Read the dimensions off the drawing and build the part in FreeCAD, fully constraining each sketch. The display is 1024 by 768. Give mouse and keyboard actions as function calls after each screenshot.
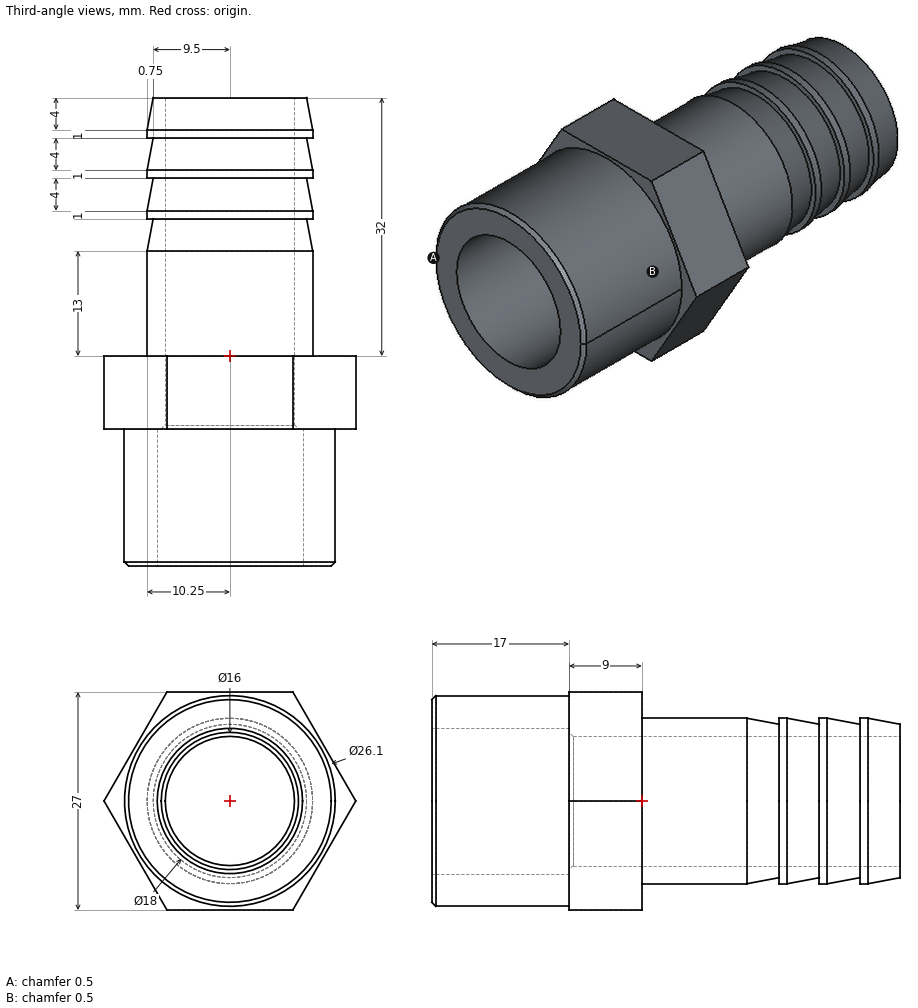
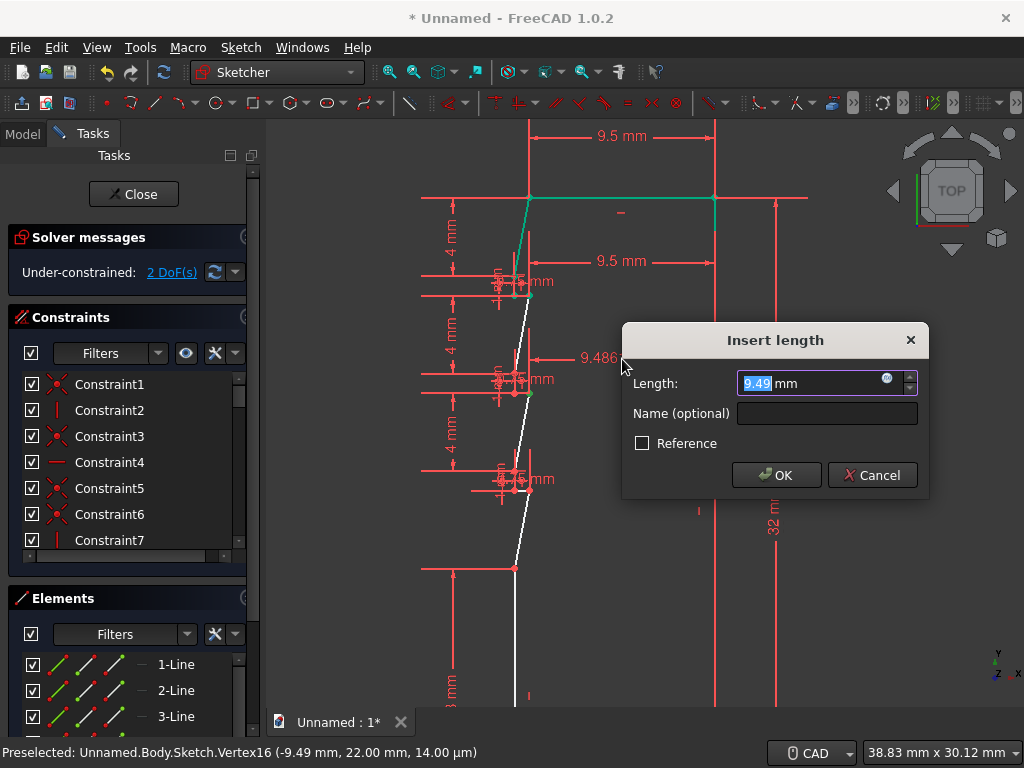
text(9.5)
key(Return)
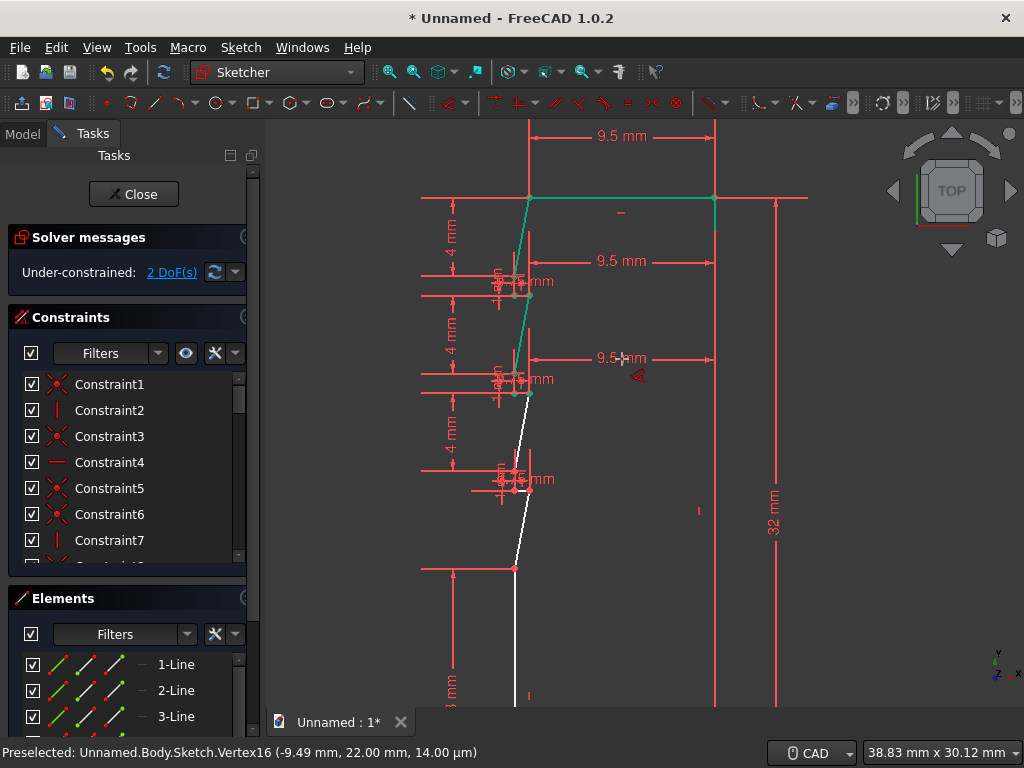
click(530, 491)
click(622, 457)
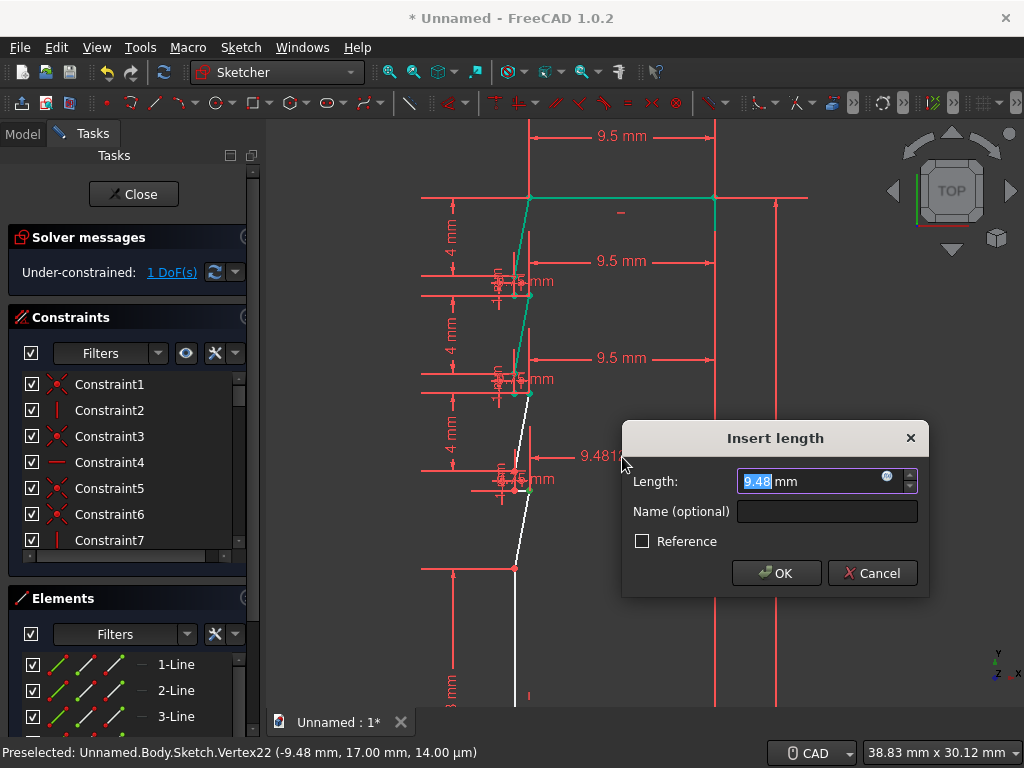
text(9.5)
key(Return)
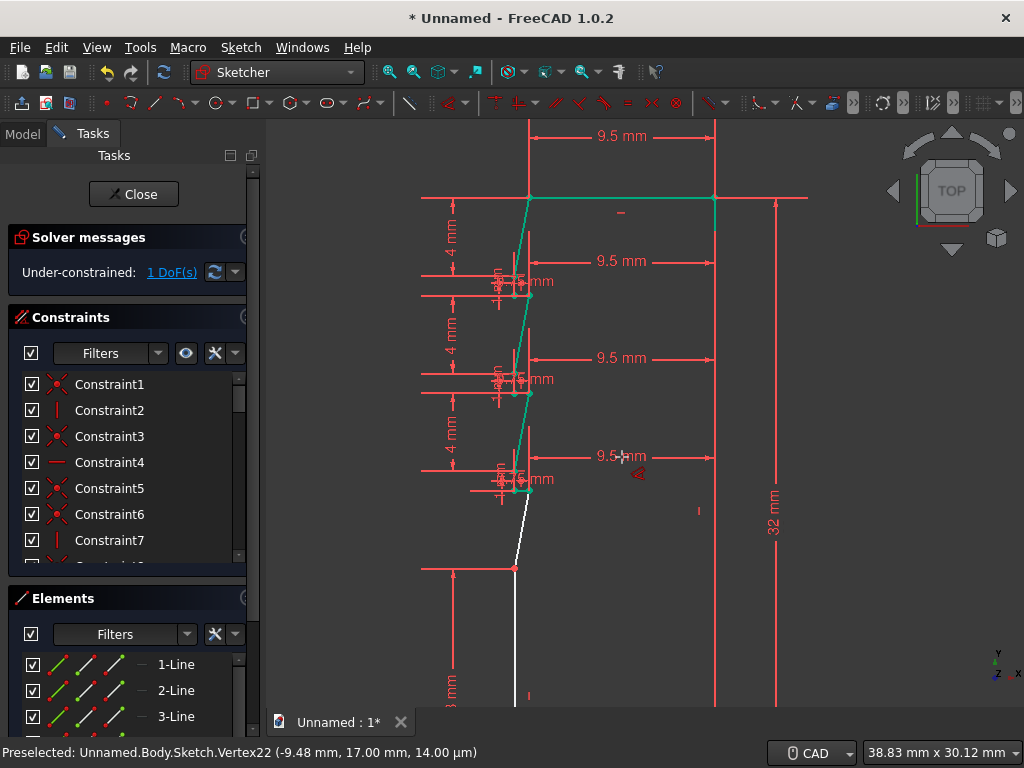
scroll(530, 295, down, 3)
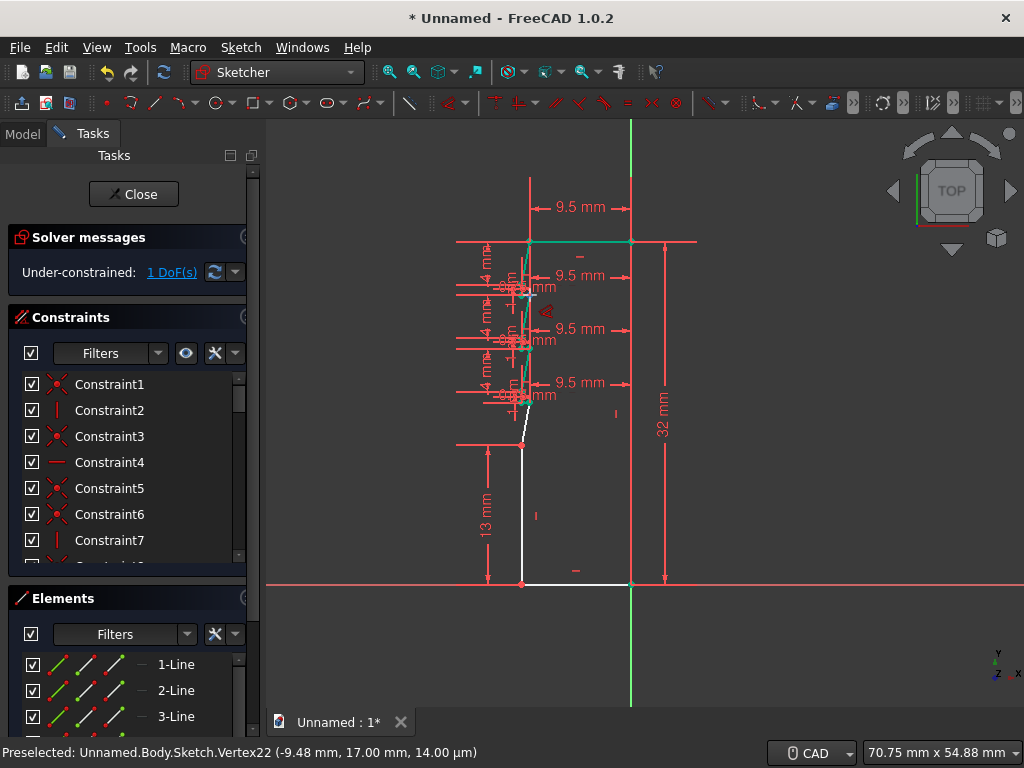
click(555, 585)
click(577, 619)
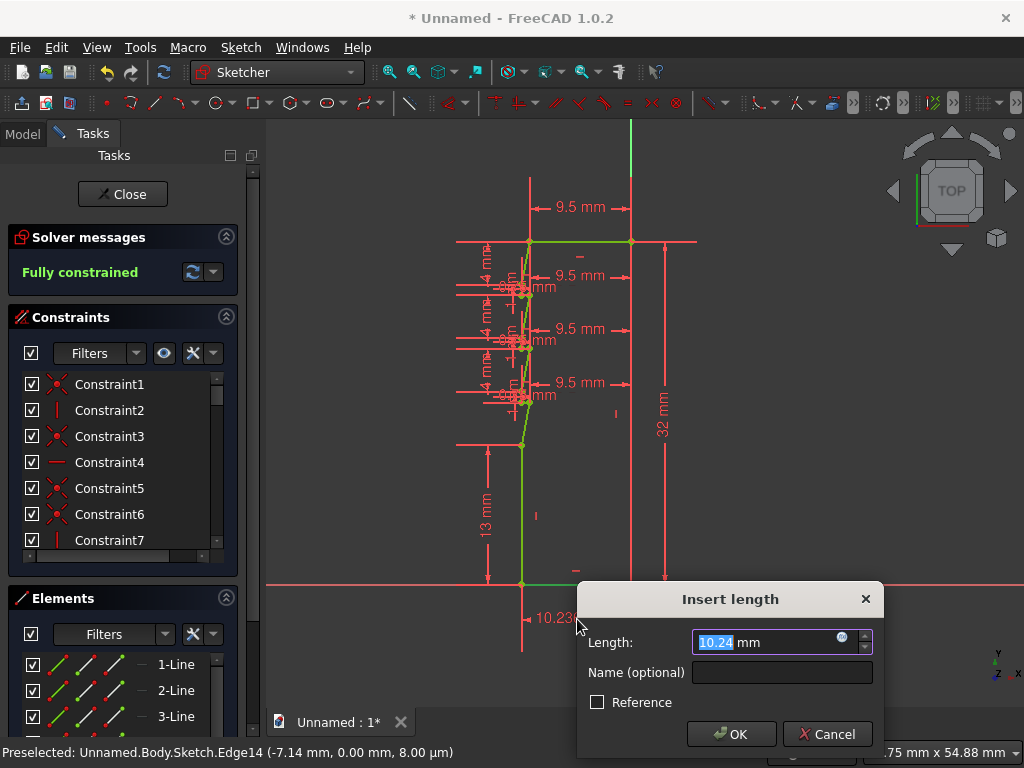
text(10.25)
key(Return)
key(Escape)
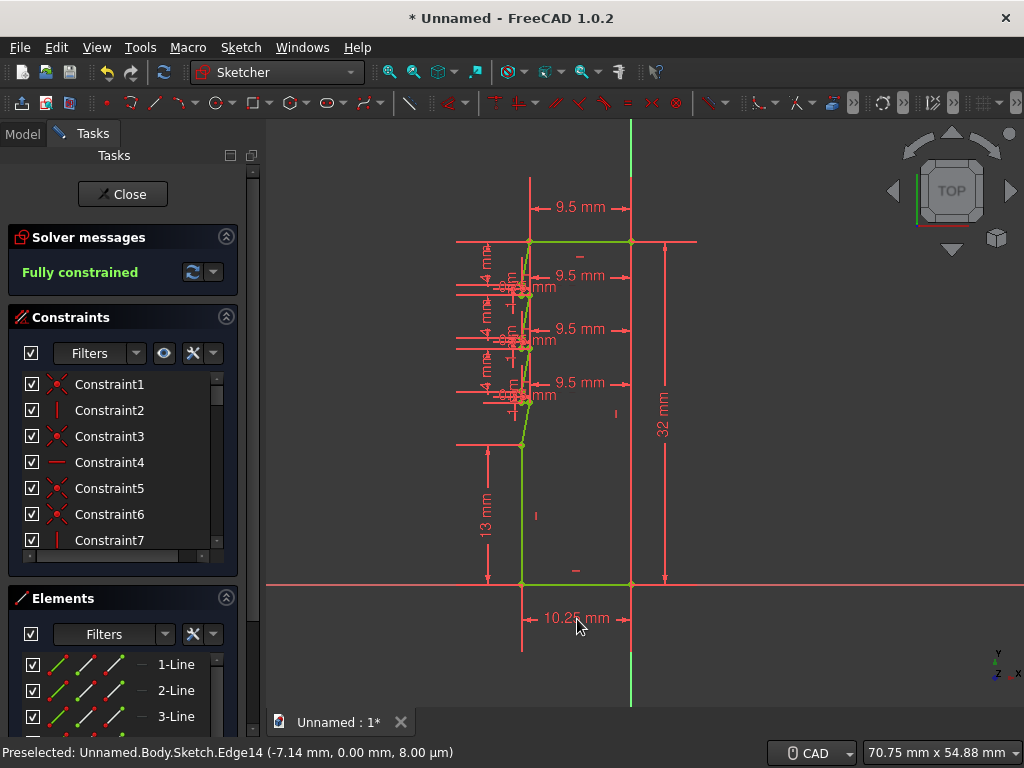
click(123, 194)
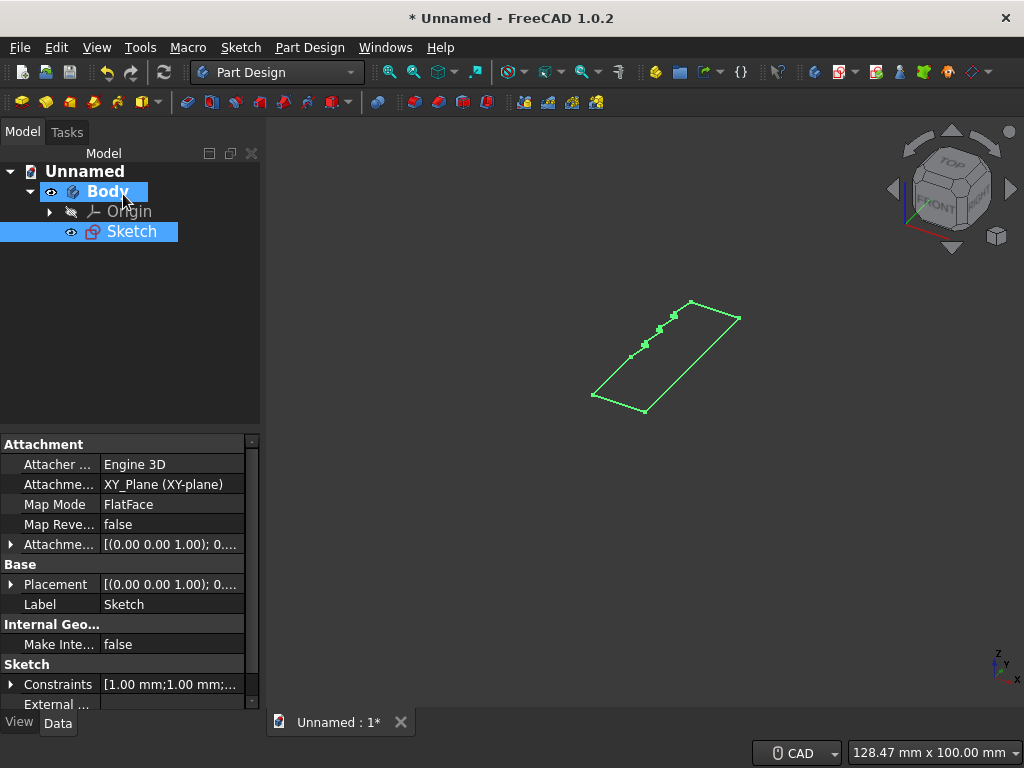
click(46, 102)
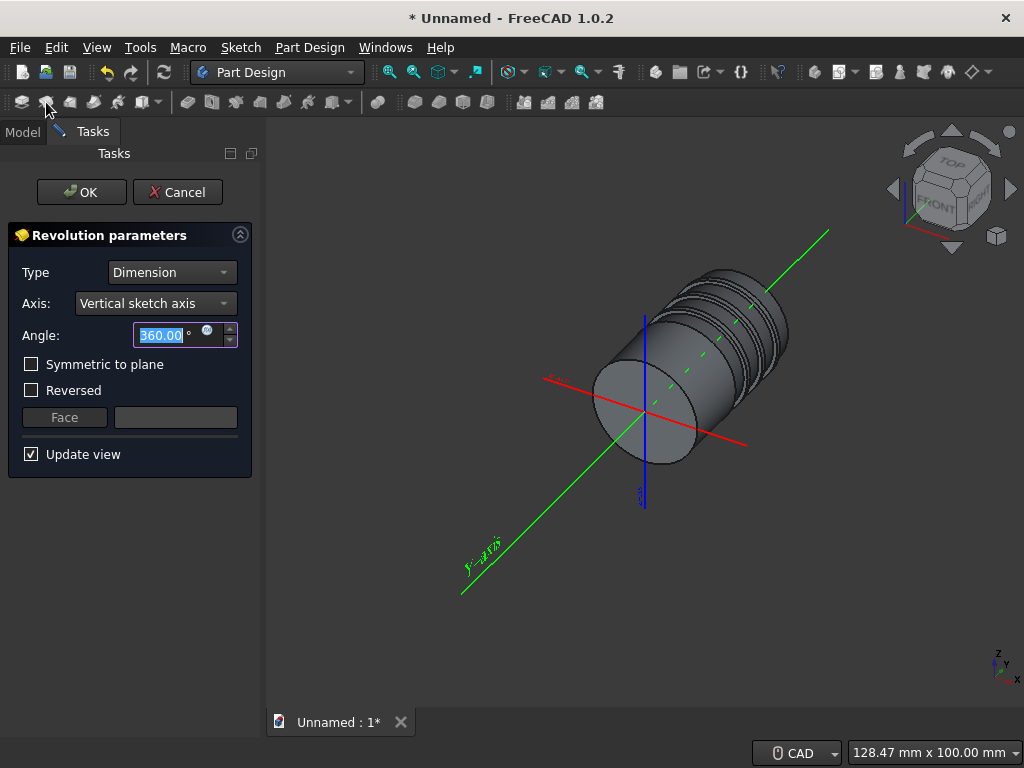
click(82, 192)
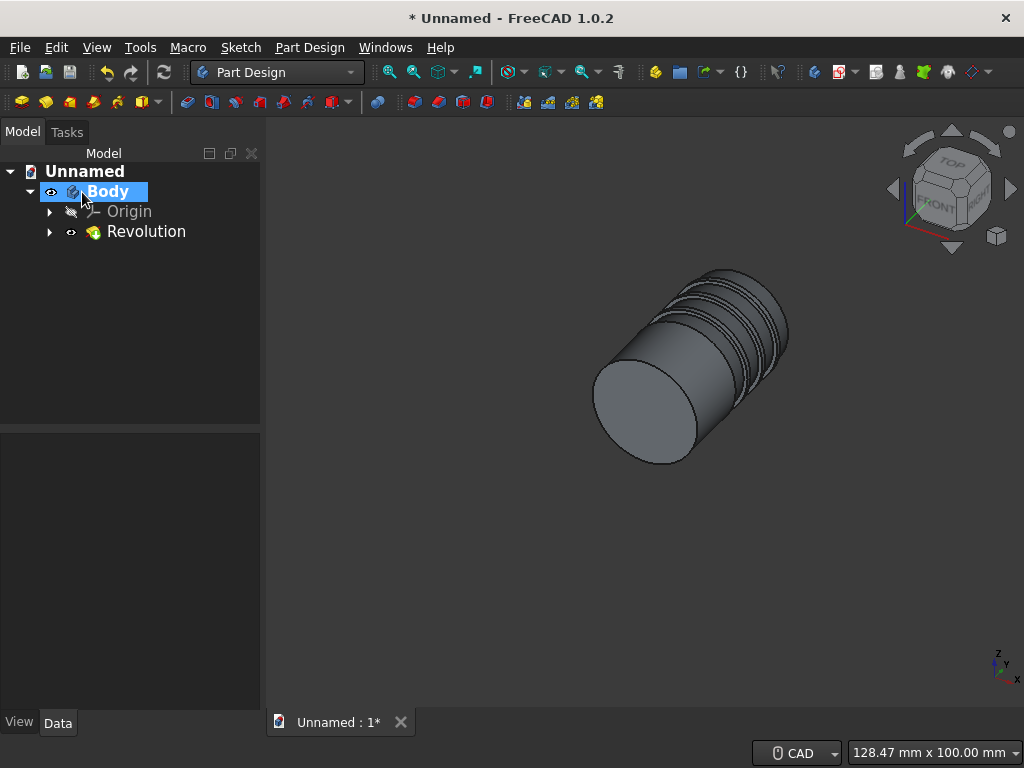
key(v)
key(f)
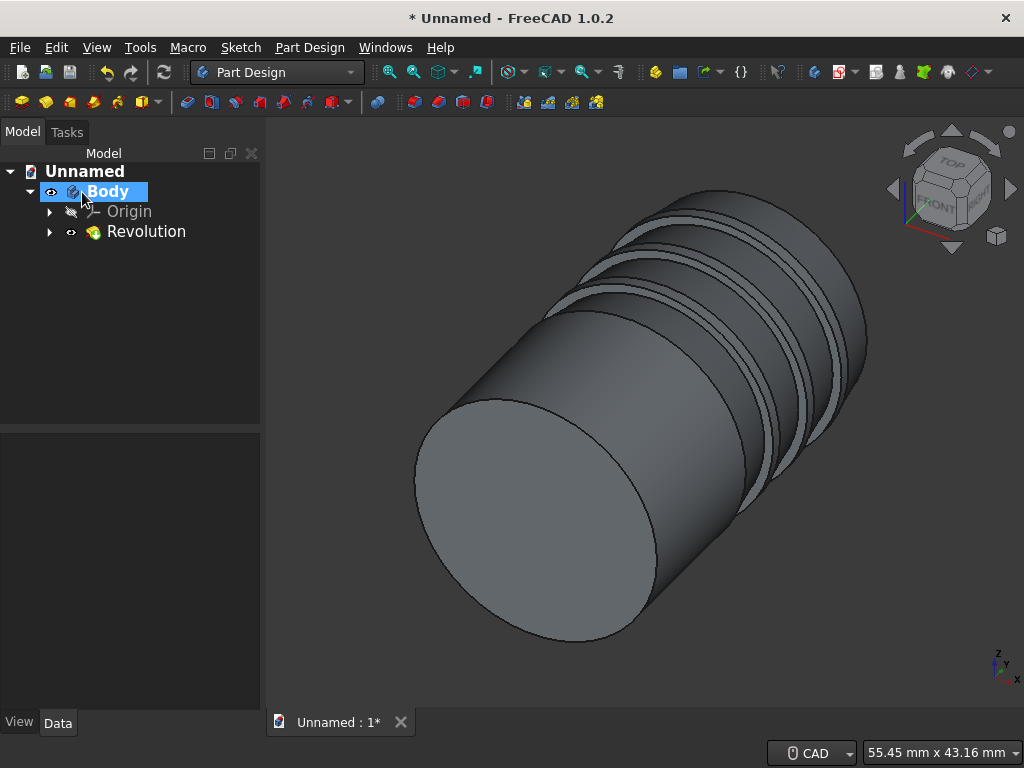
click(536, 520)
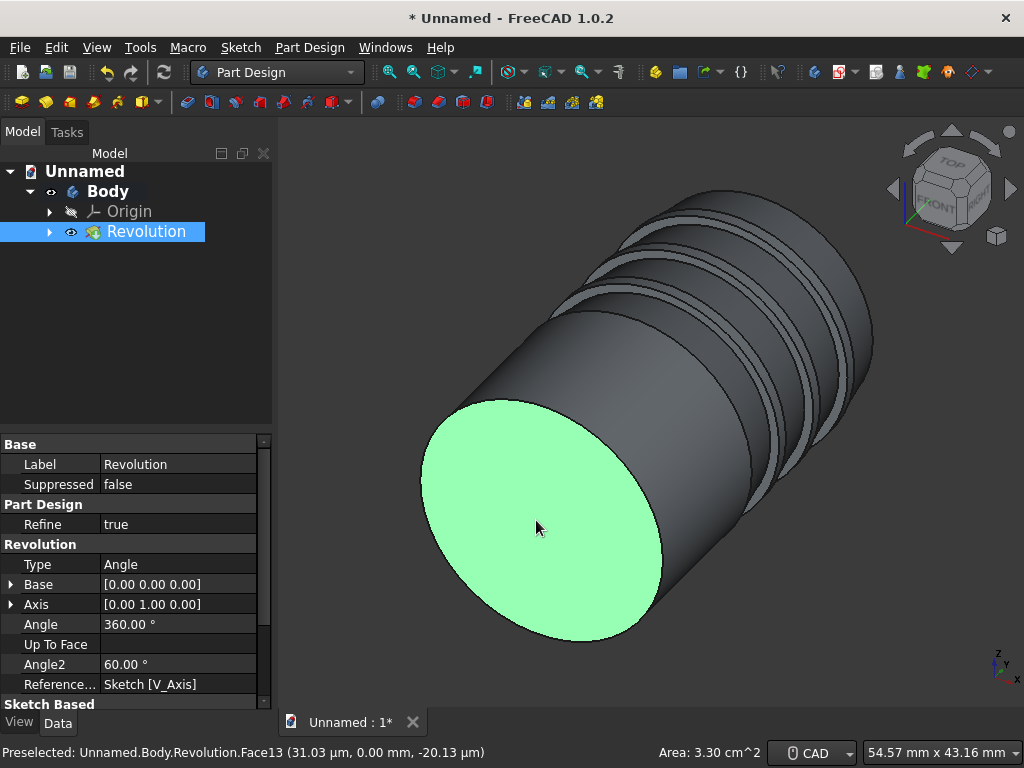
click(840, 72)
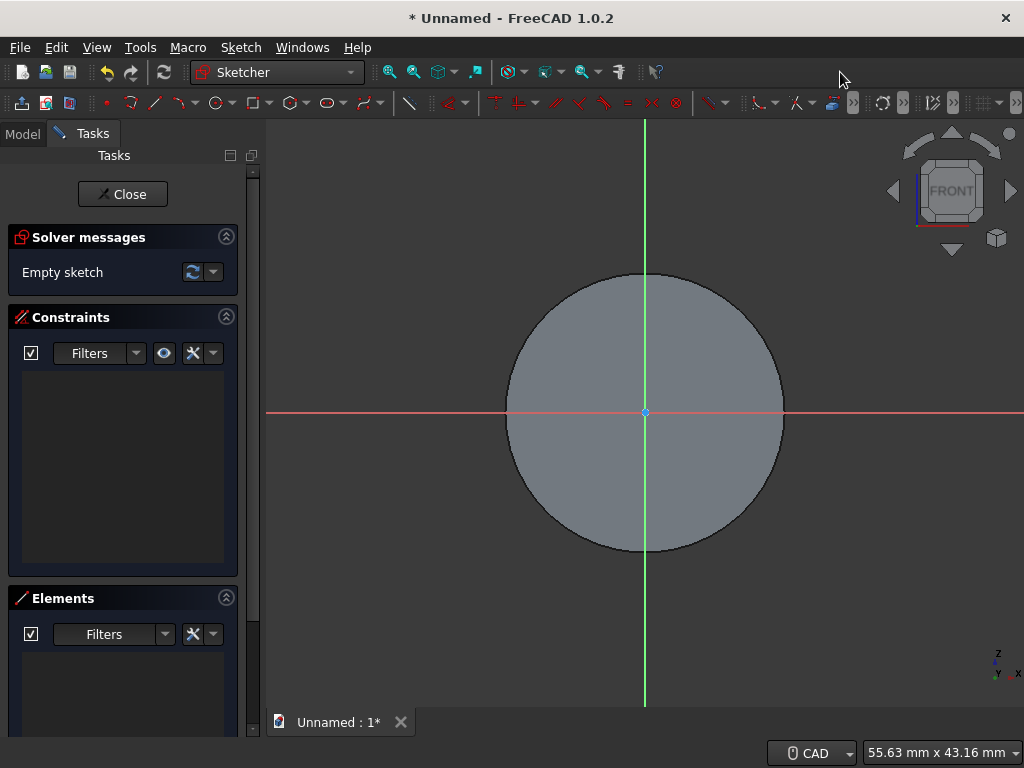
scroll(294, 413, down, 1)